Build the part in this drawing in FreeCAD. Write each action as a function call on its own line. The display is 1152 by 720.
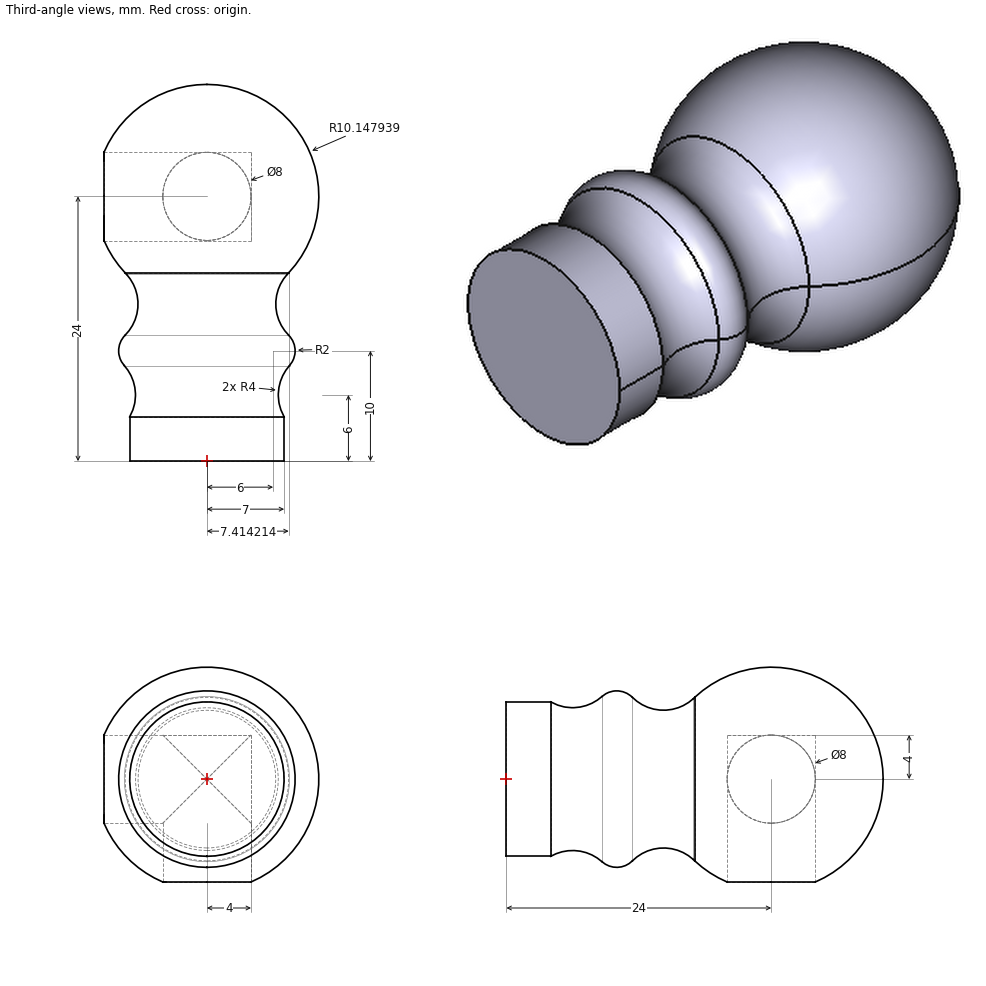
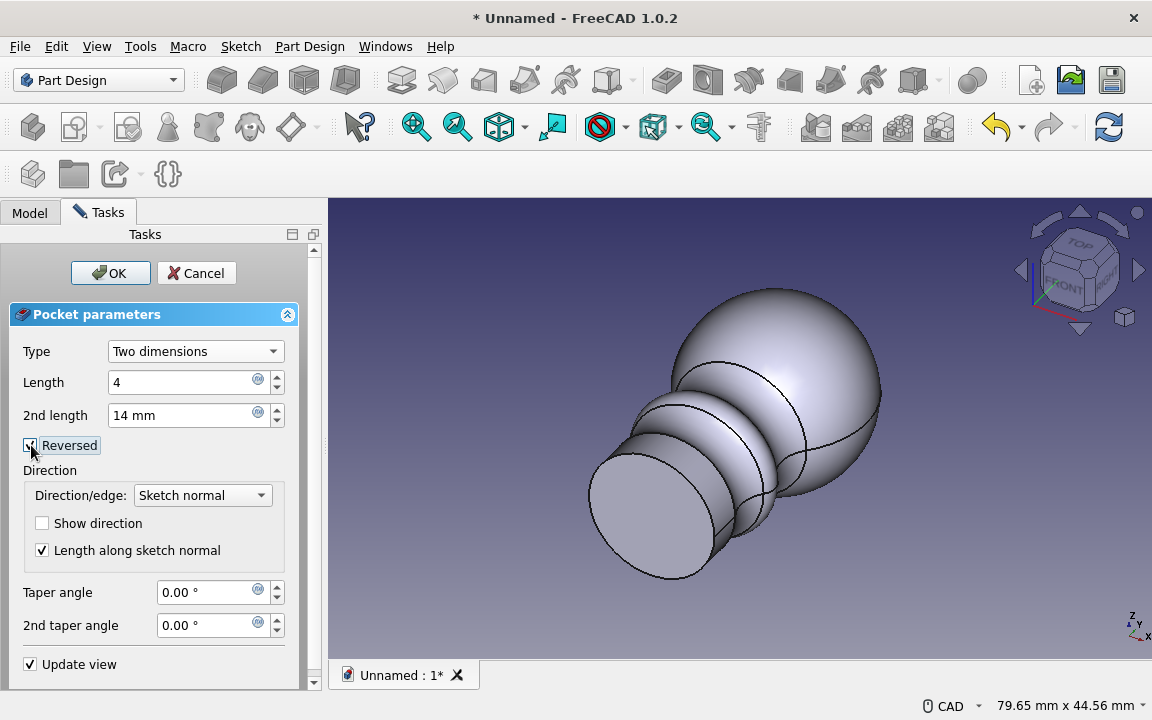
click(111, 273)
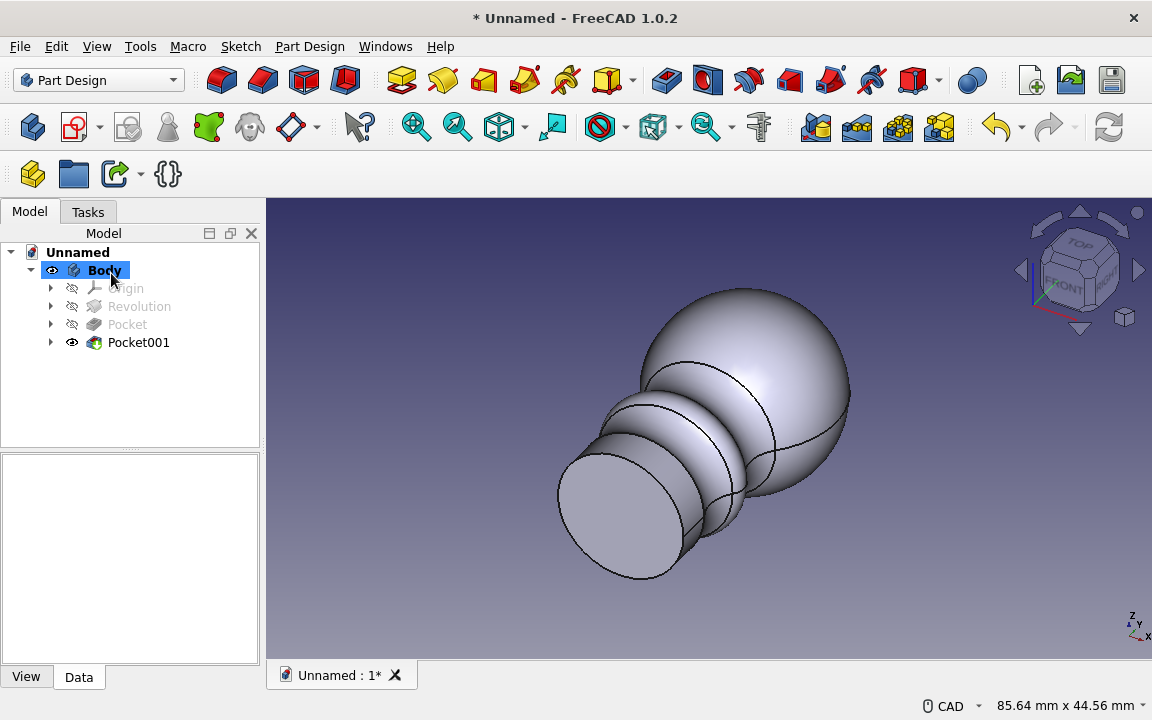
key(0)